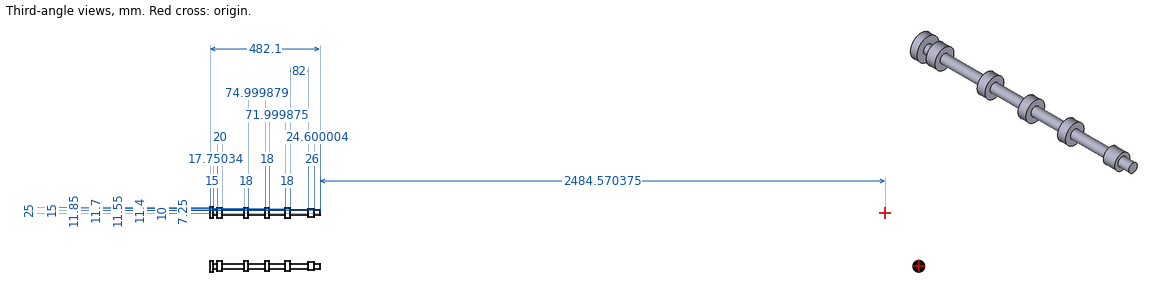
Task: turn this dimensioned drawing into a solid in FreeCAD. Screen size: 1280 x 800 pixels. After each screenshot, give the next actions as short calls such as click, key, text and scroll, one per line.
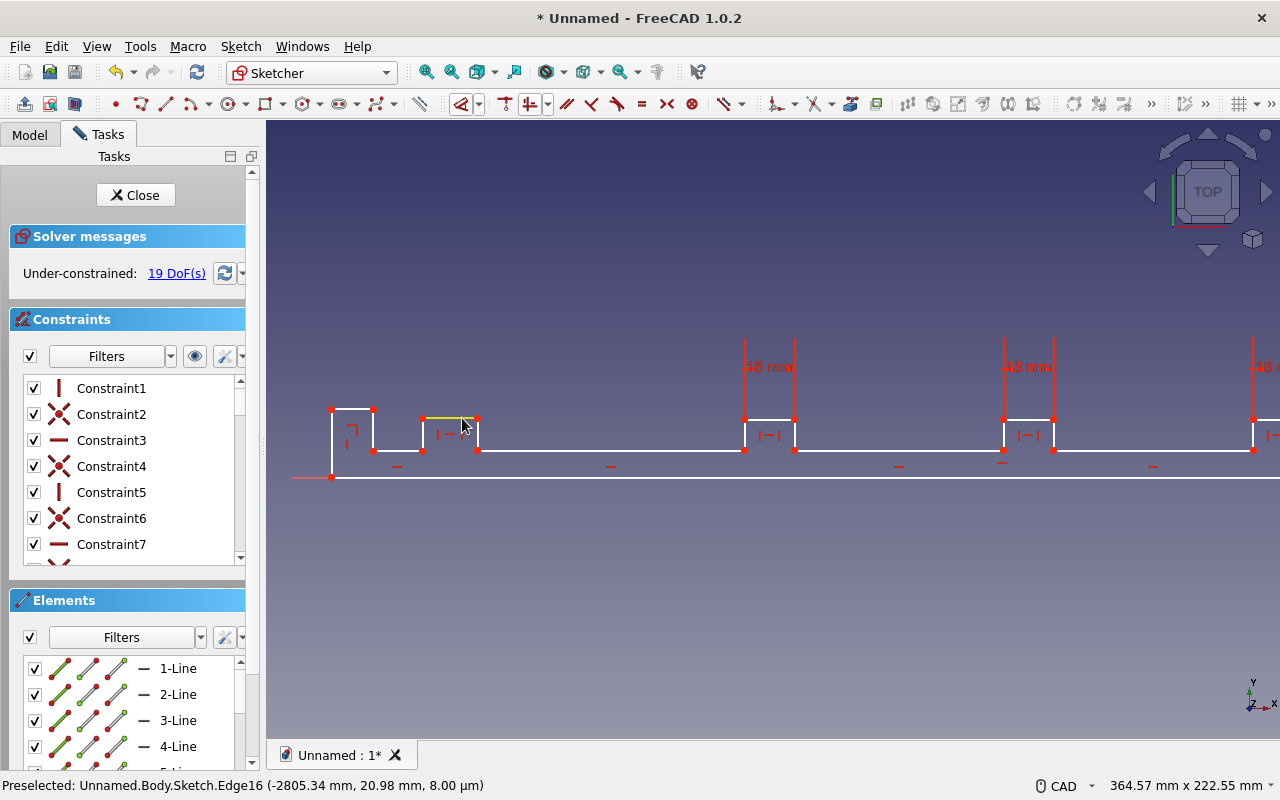
click(461, 418)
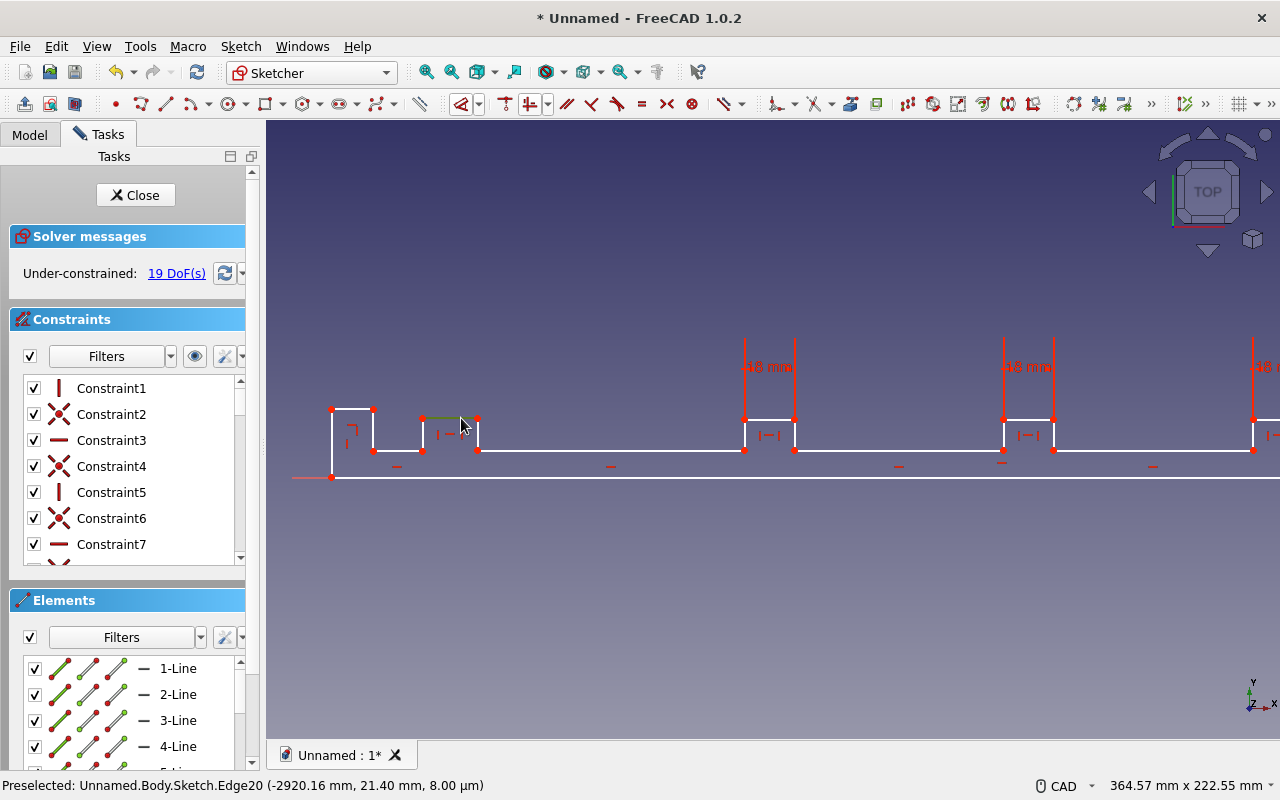
click(478, 104)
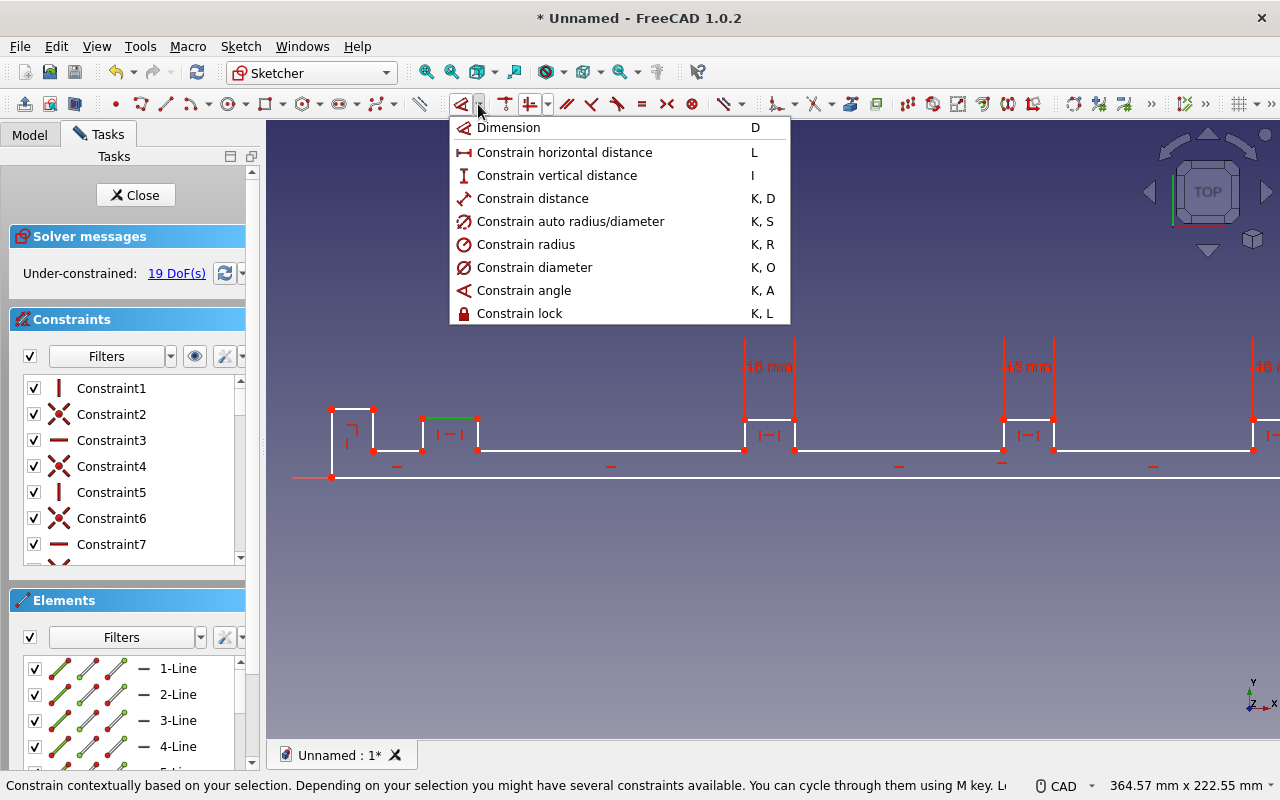
click(620, 152)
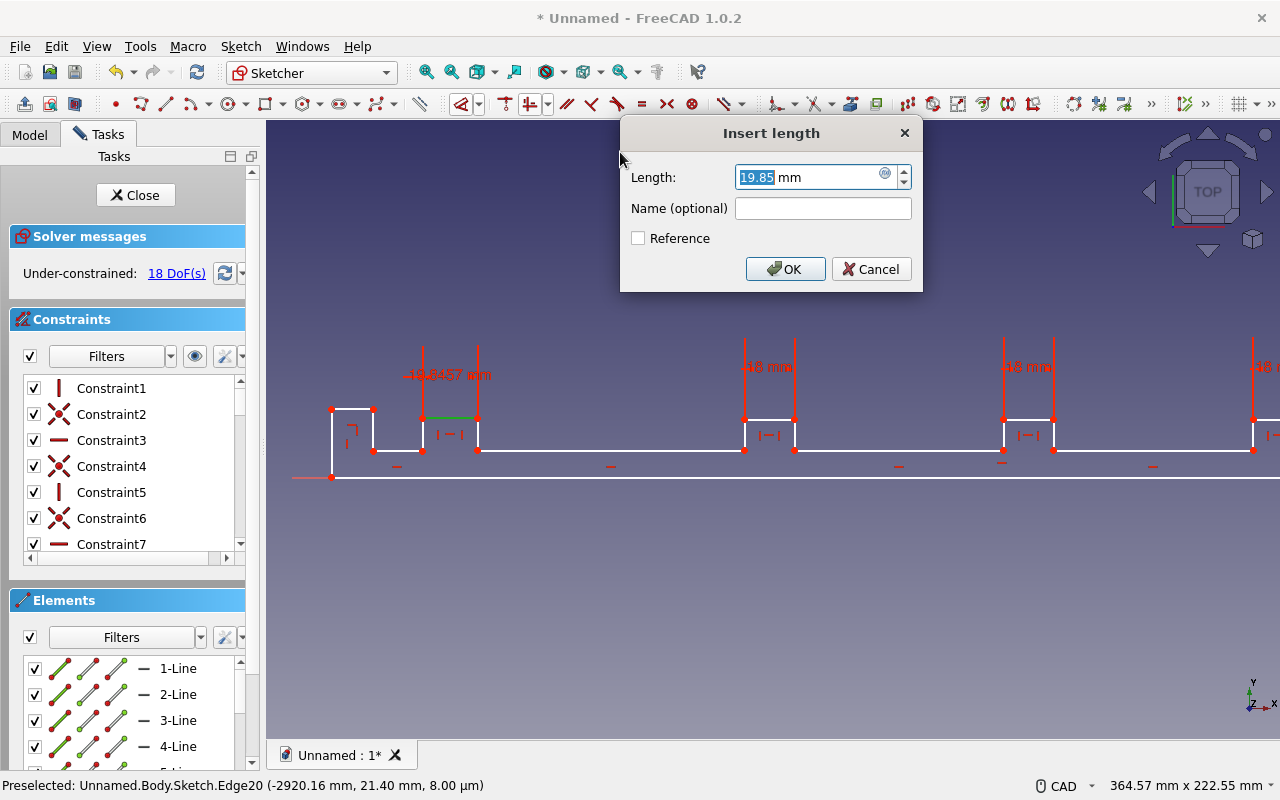
text(20)
key(Return)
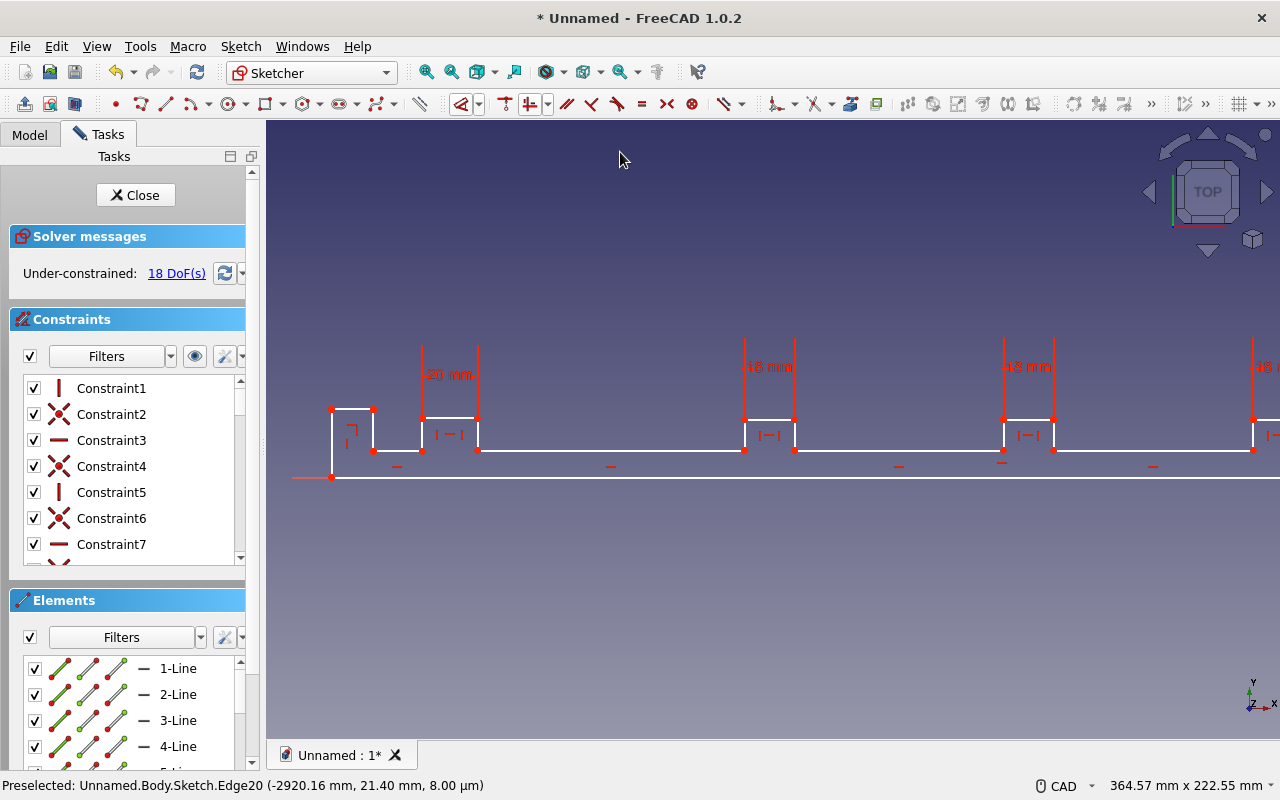
click(373, 439)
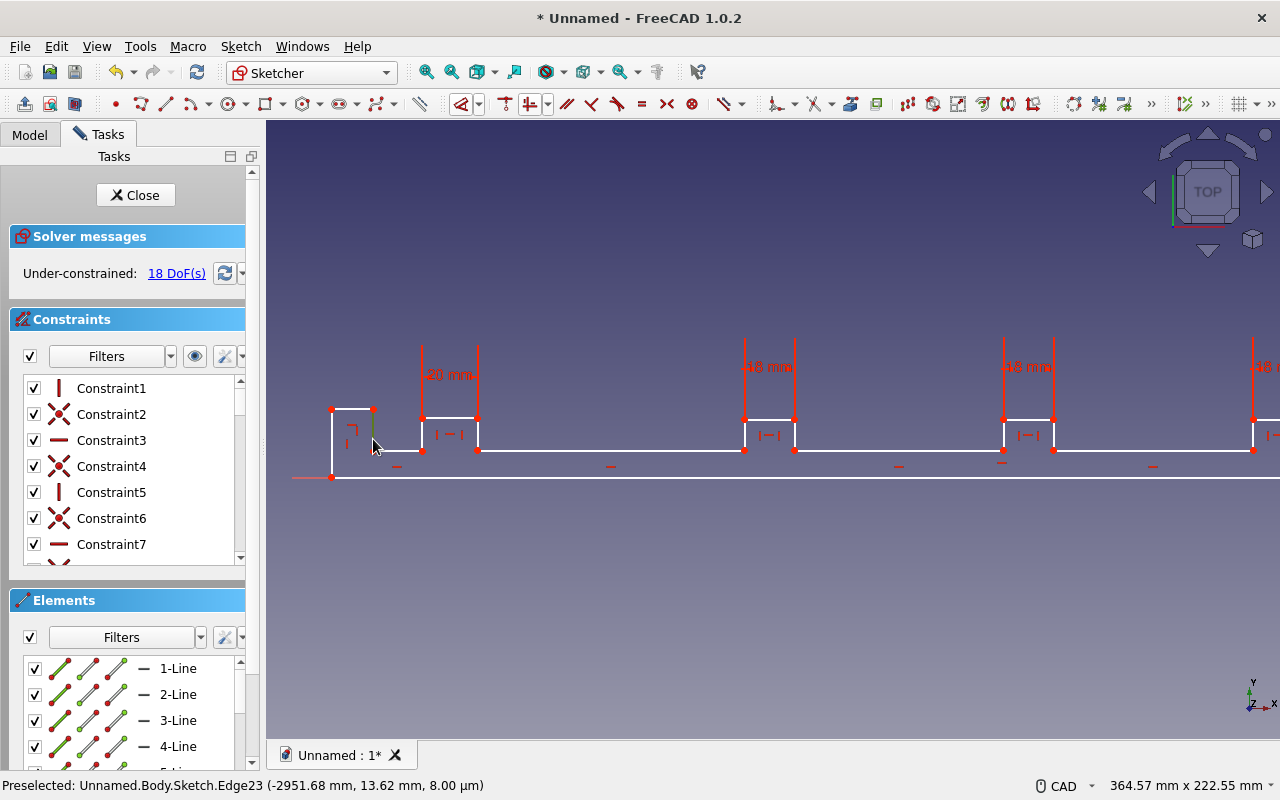
key(i)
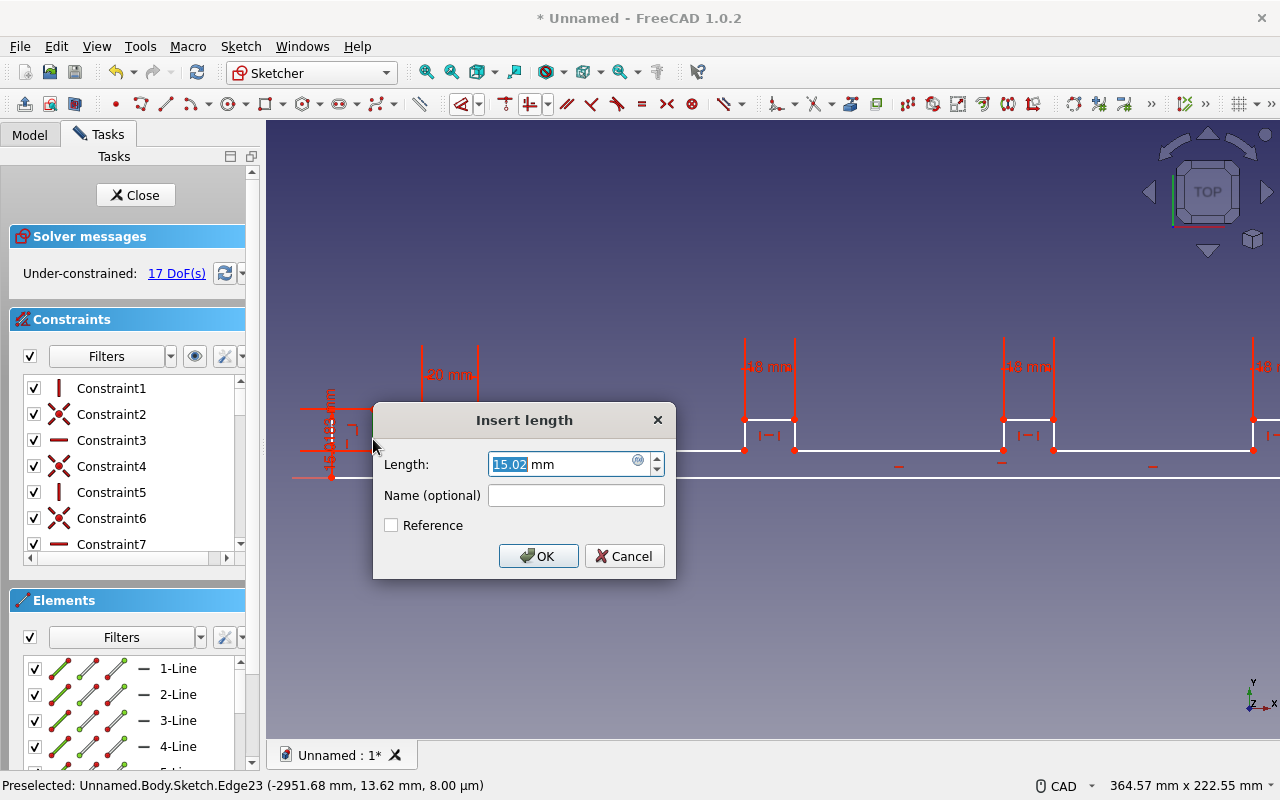
text(15)
key(Return)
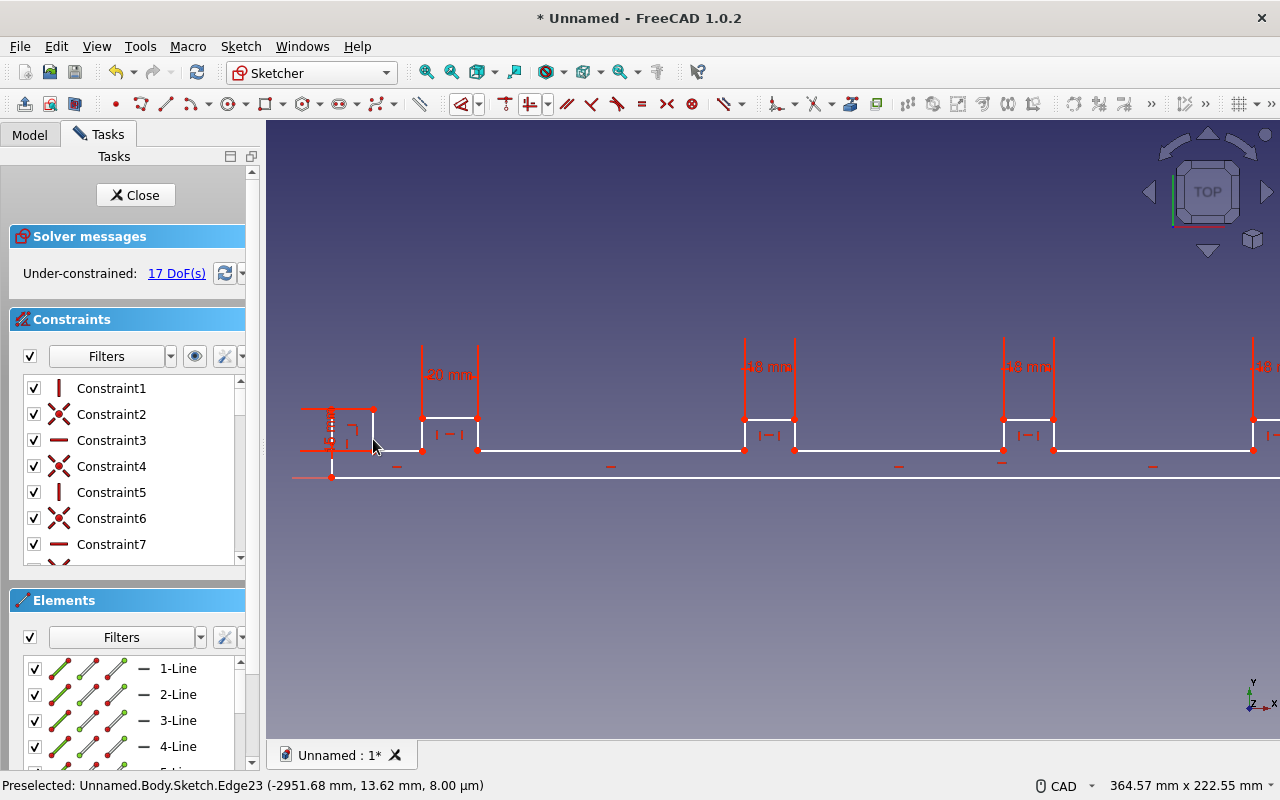
click(361, 409)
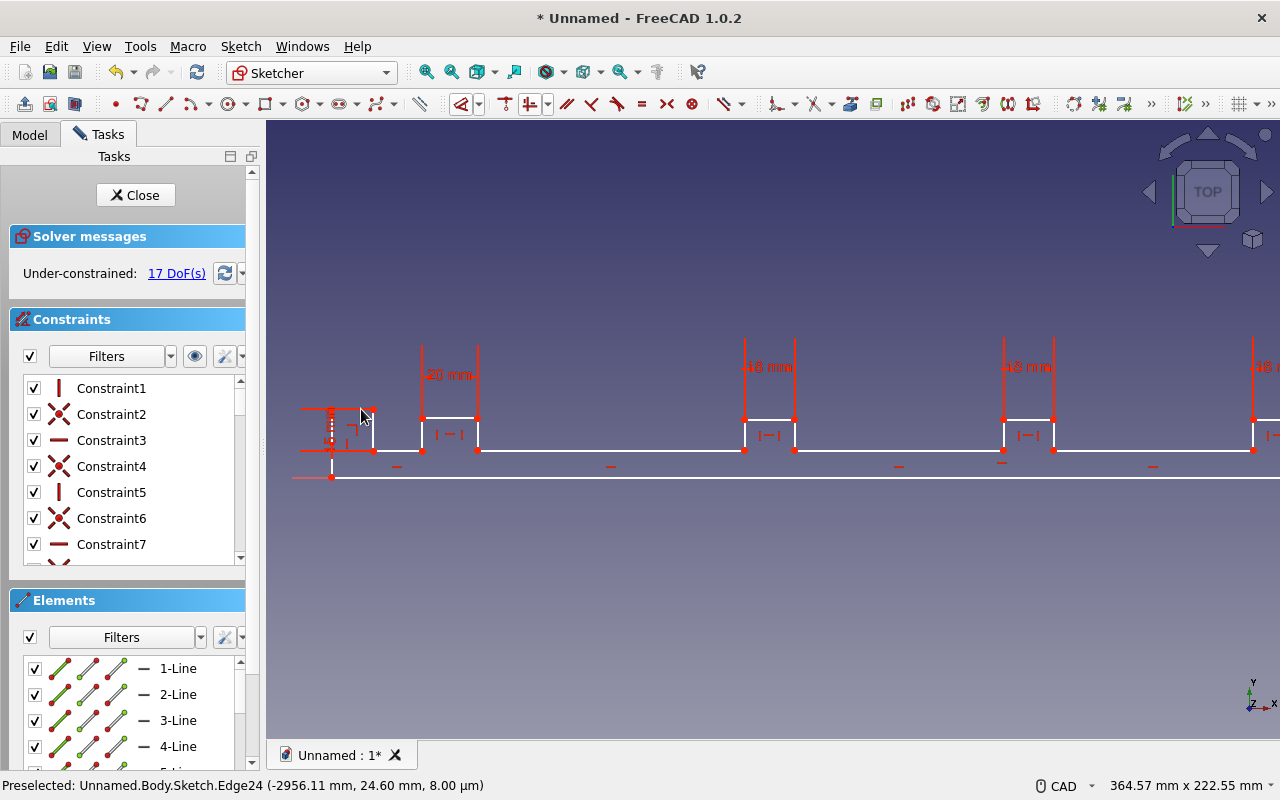
click(478, 104)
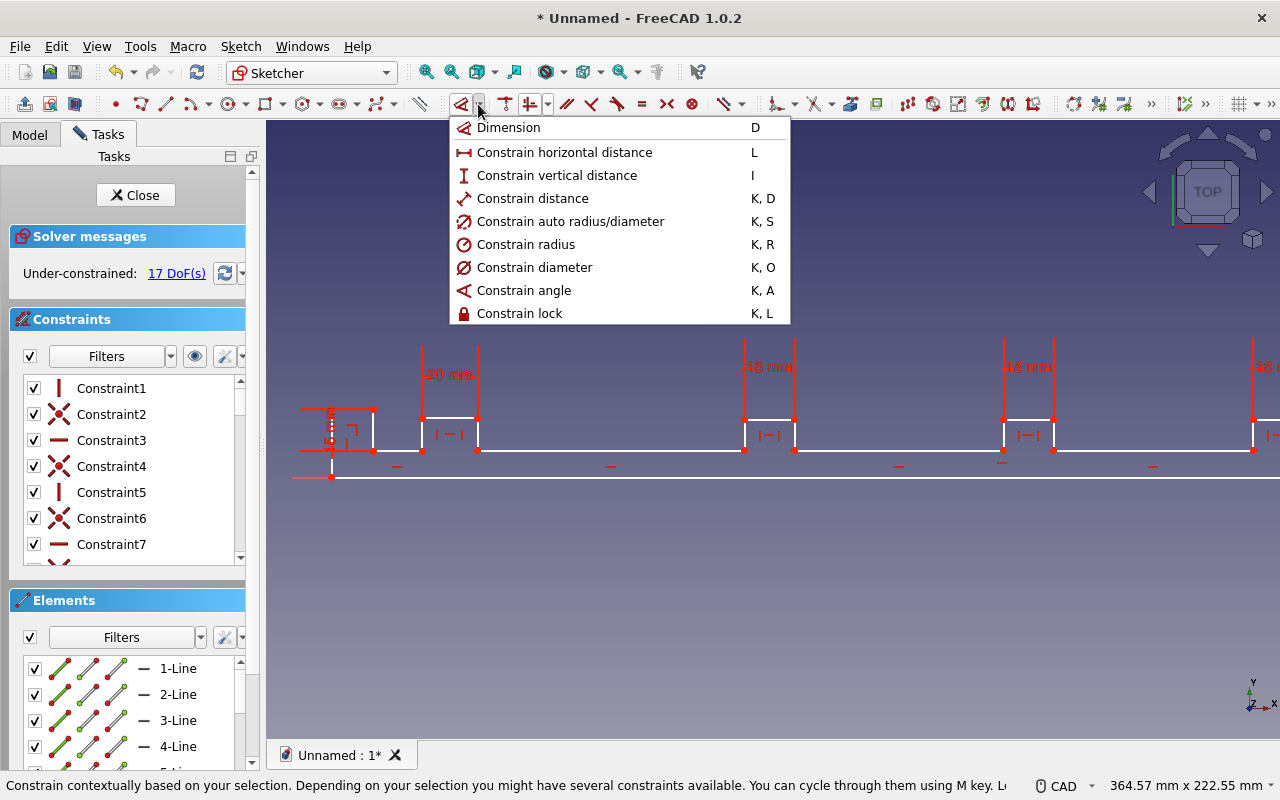
click(620, 152)